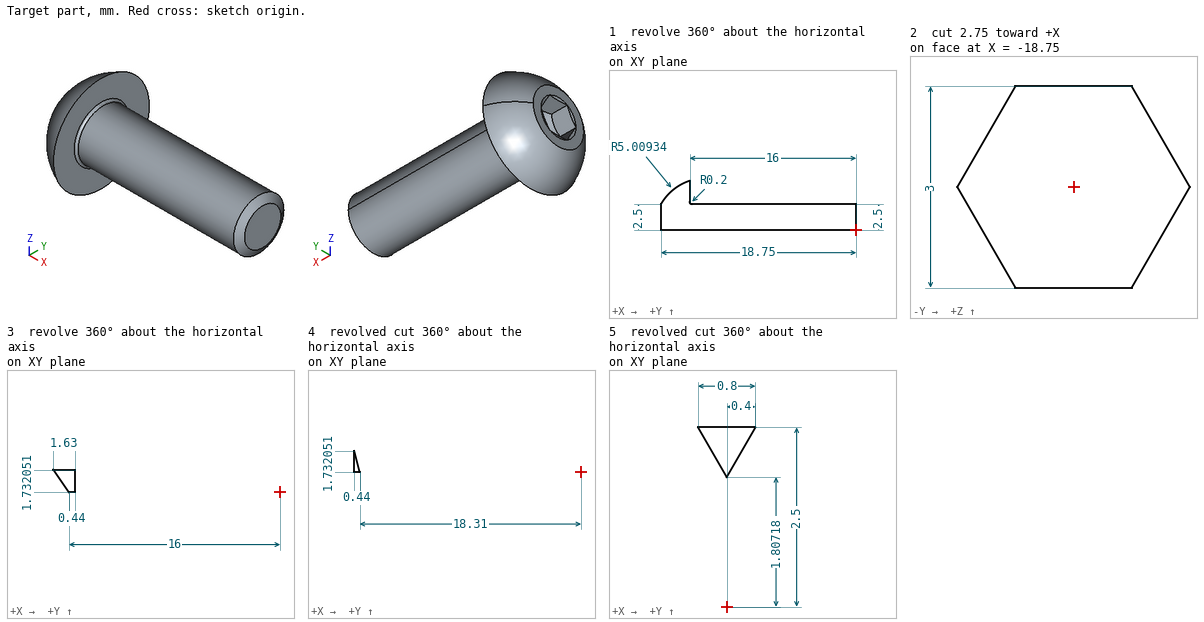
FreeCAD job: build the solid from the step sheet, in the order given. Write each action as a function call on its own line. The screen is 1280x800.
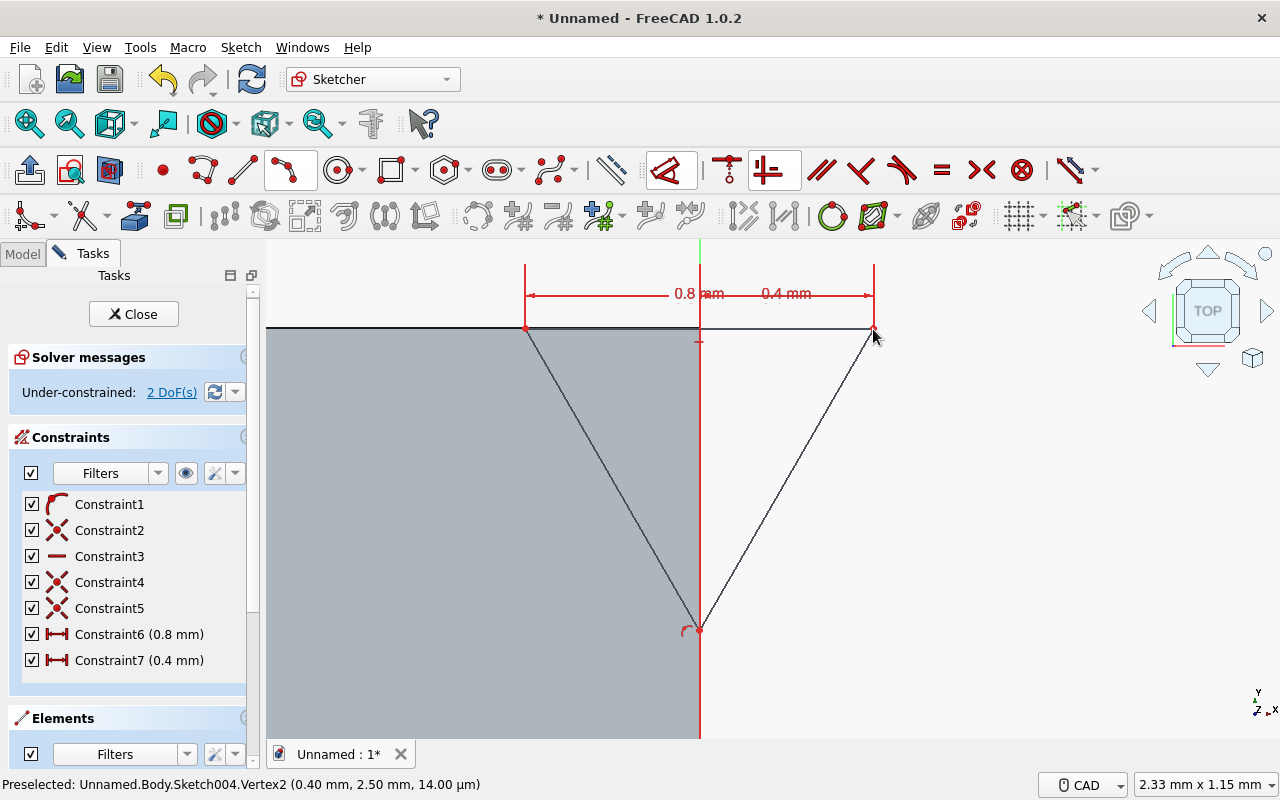
click(874, 329)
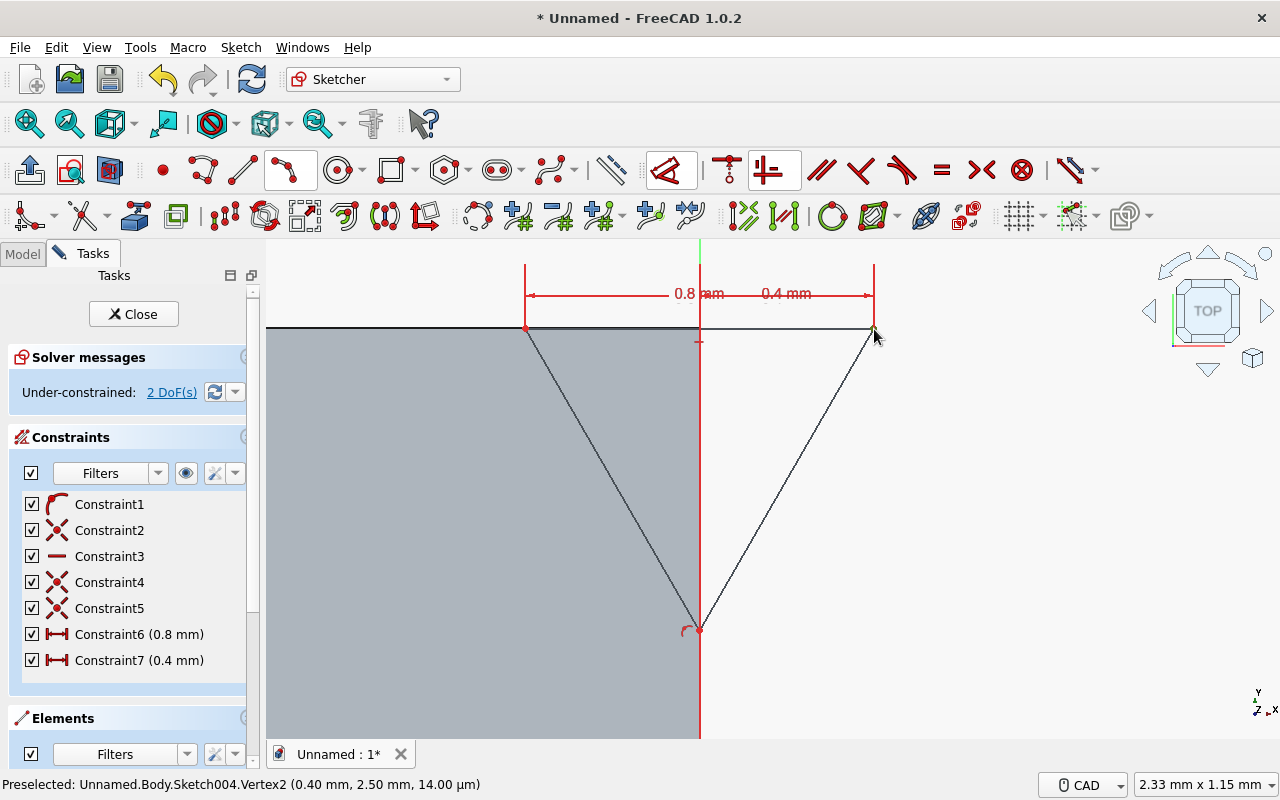
key(i)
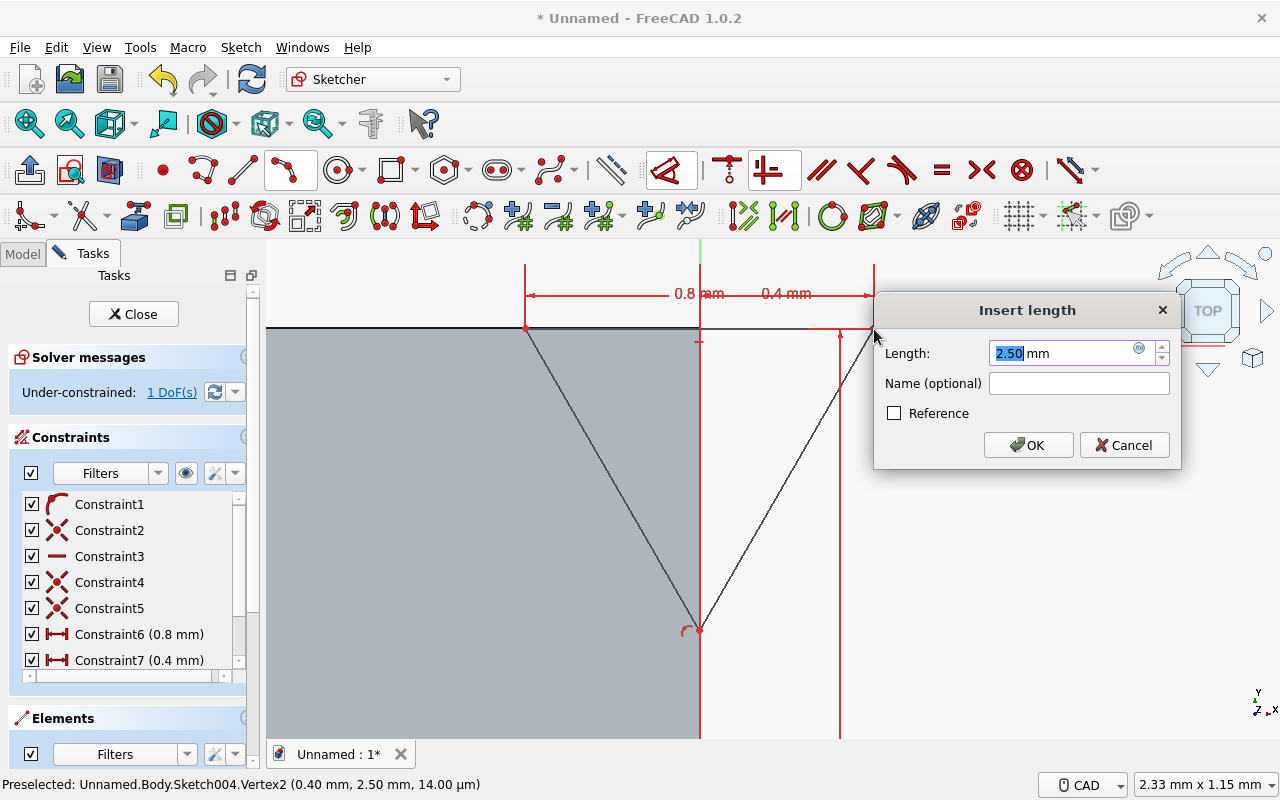
text(2.5)
key(Return)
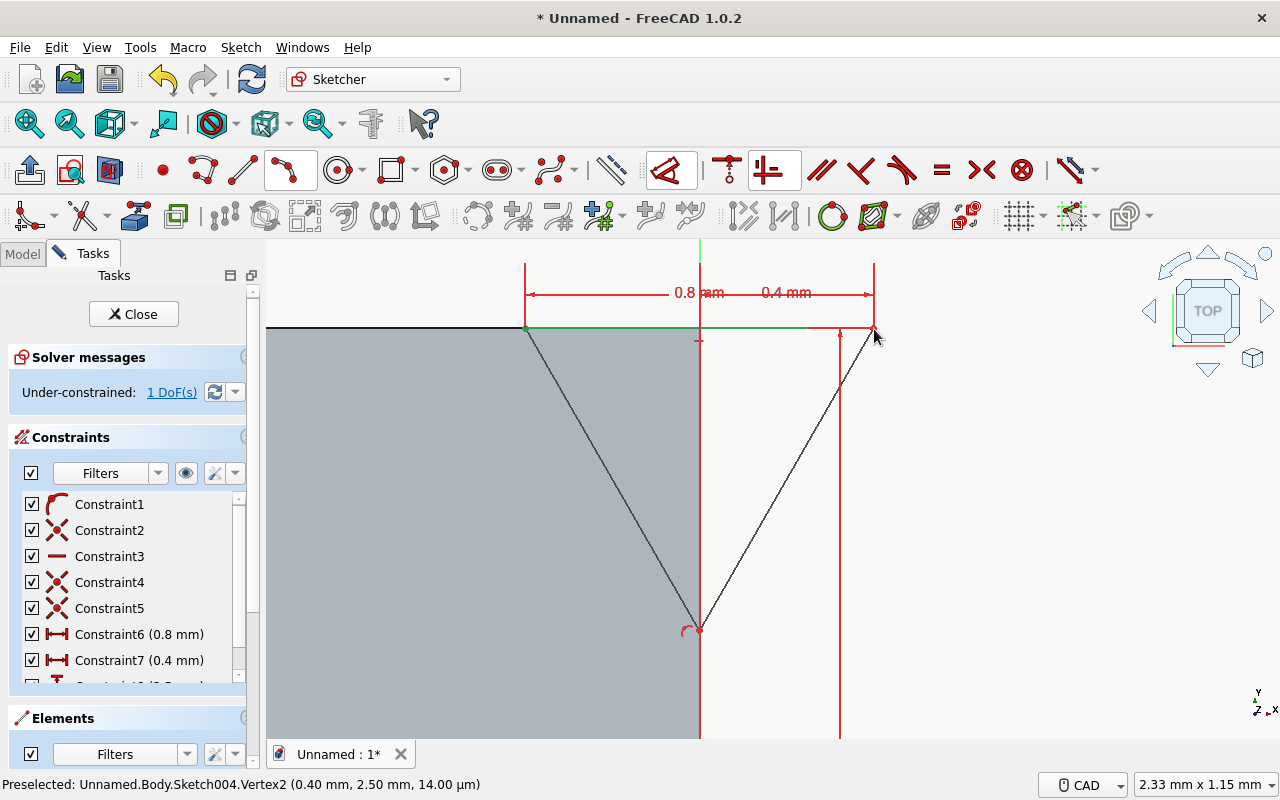
click(700, 631)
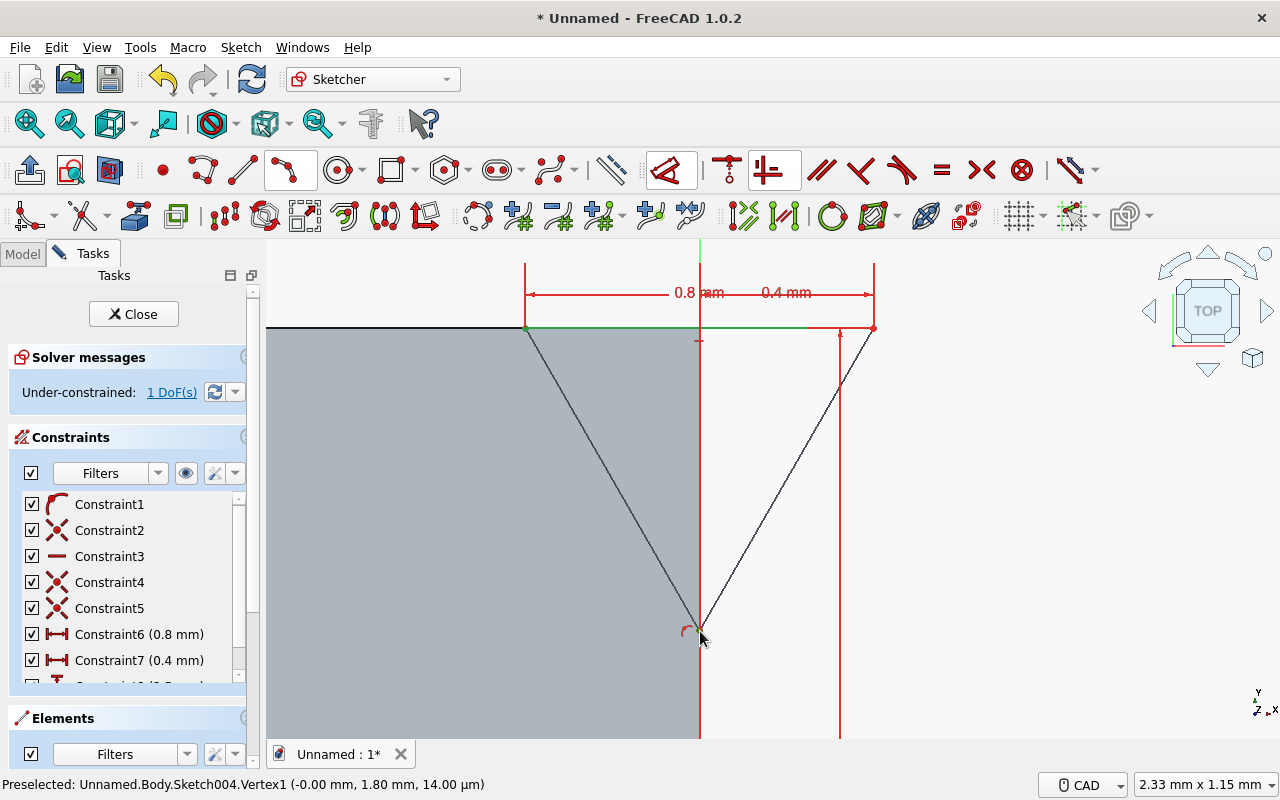
click(692, 170)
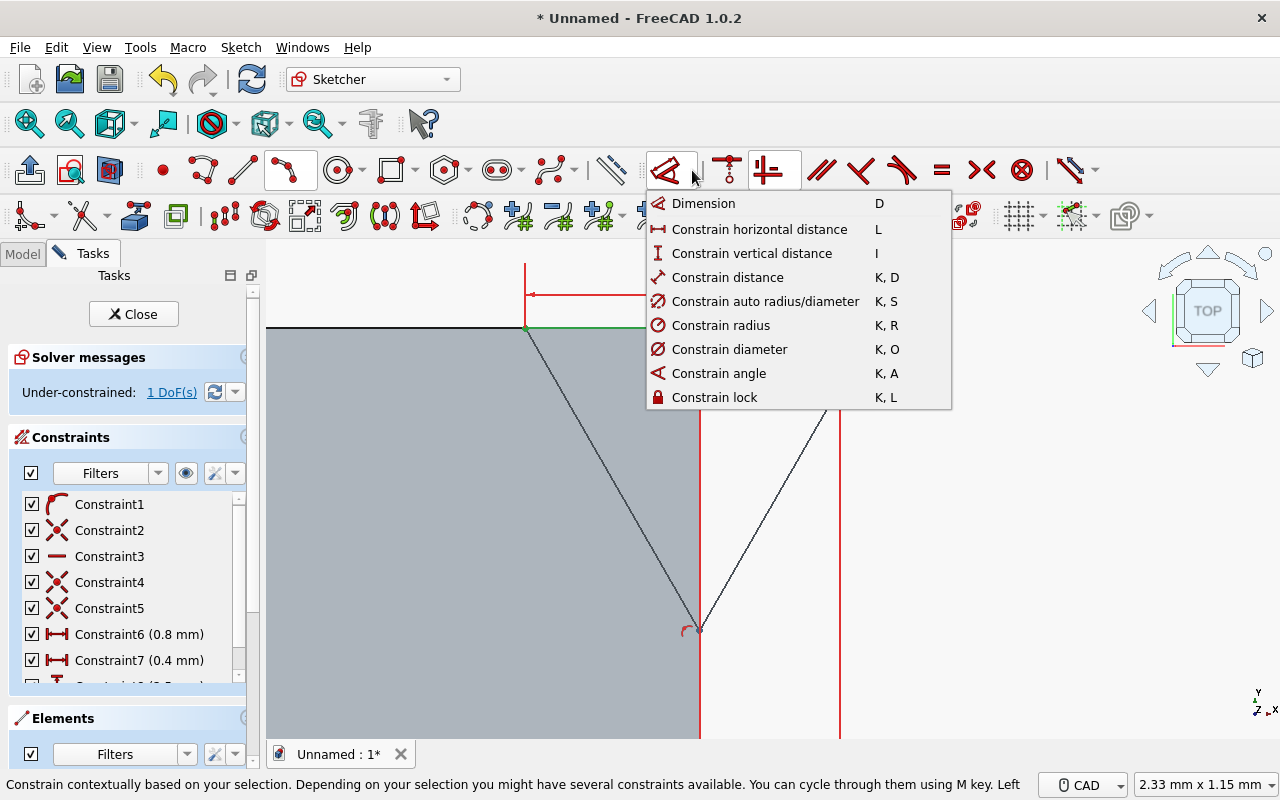
click(799, 253)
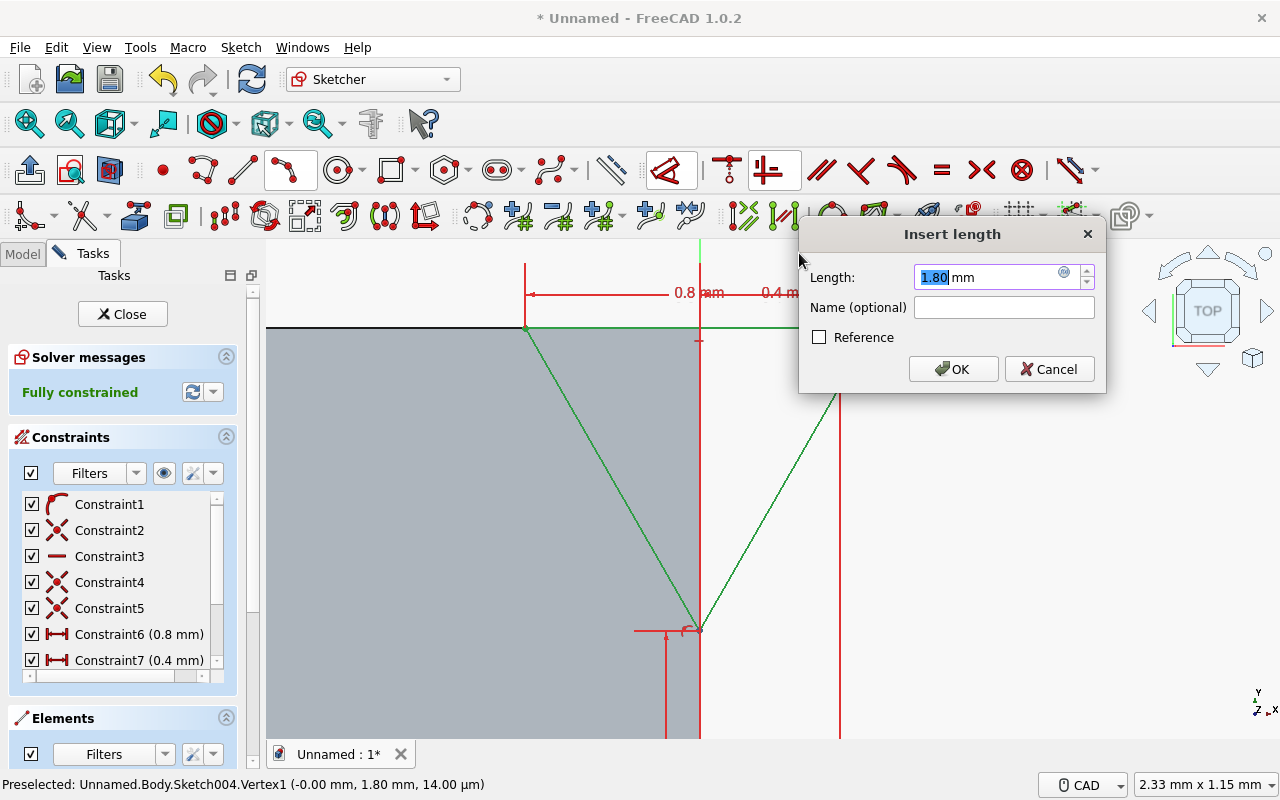
text(1.80718)
key(Return)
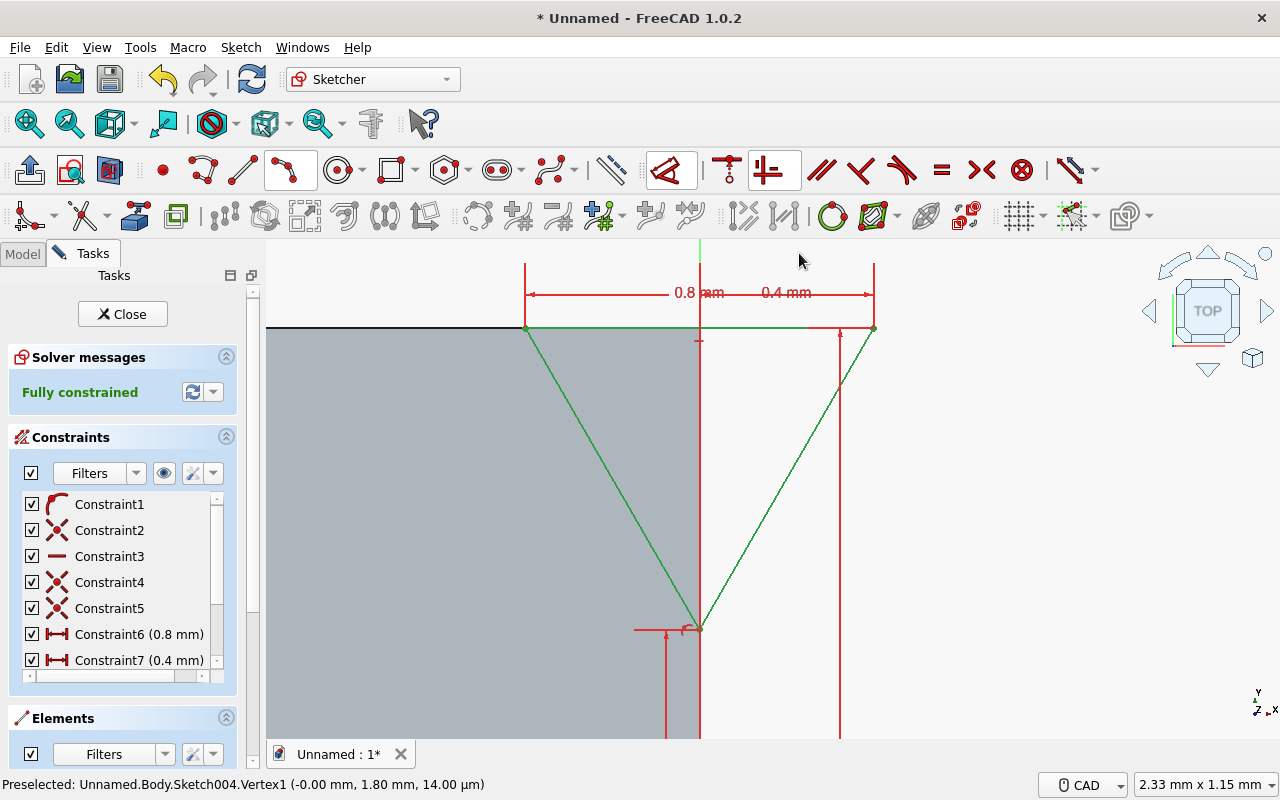
click(123, 314)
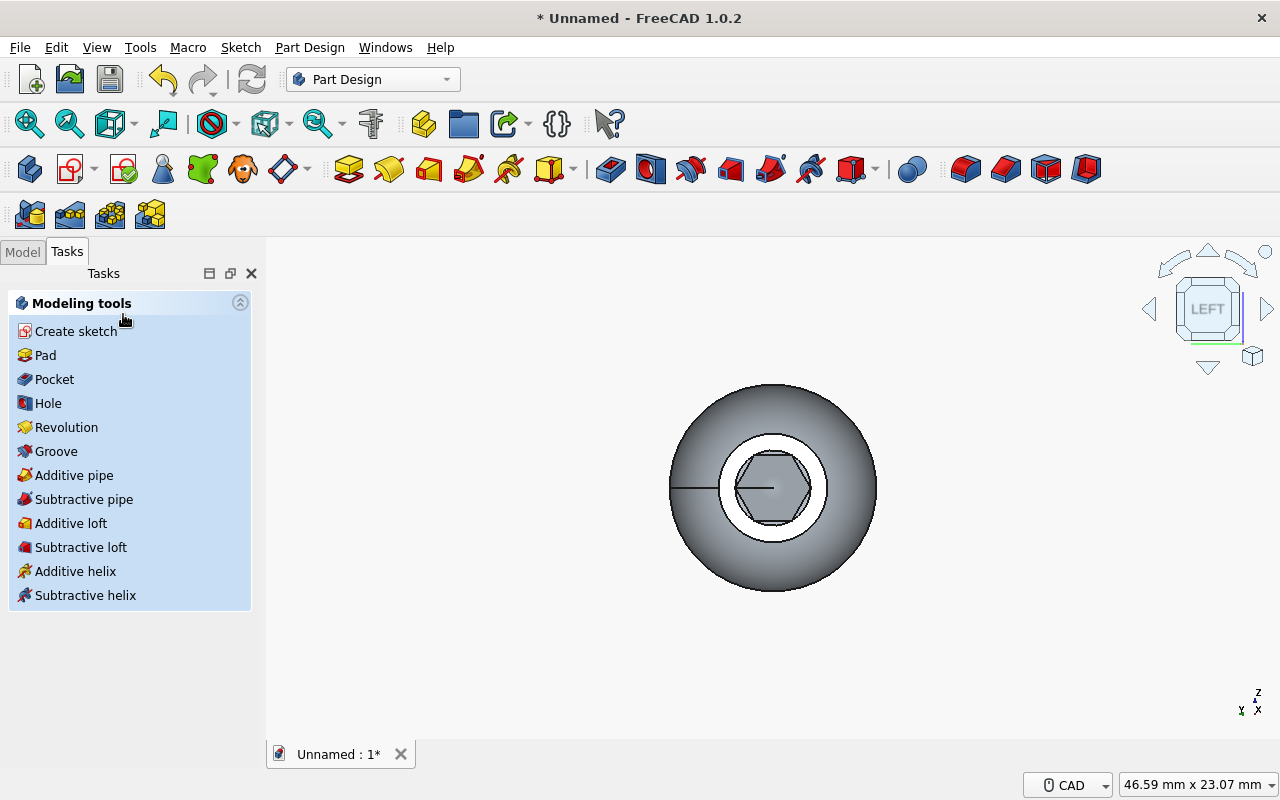
click(692, 170)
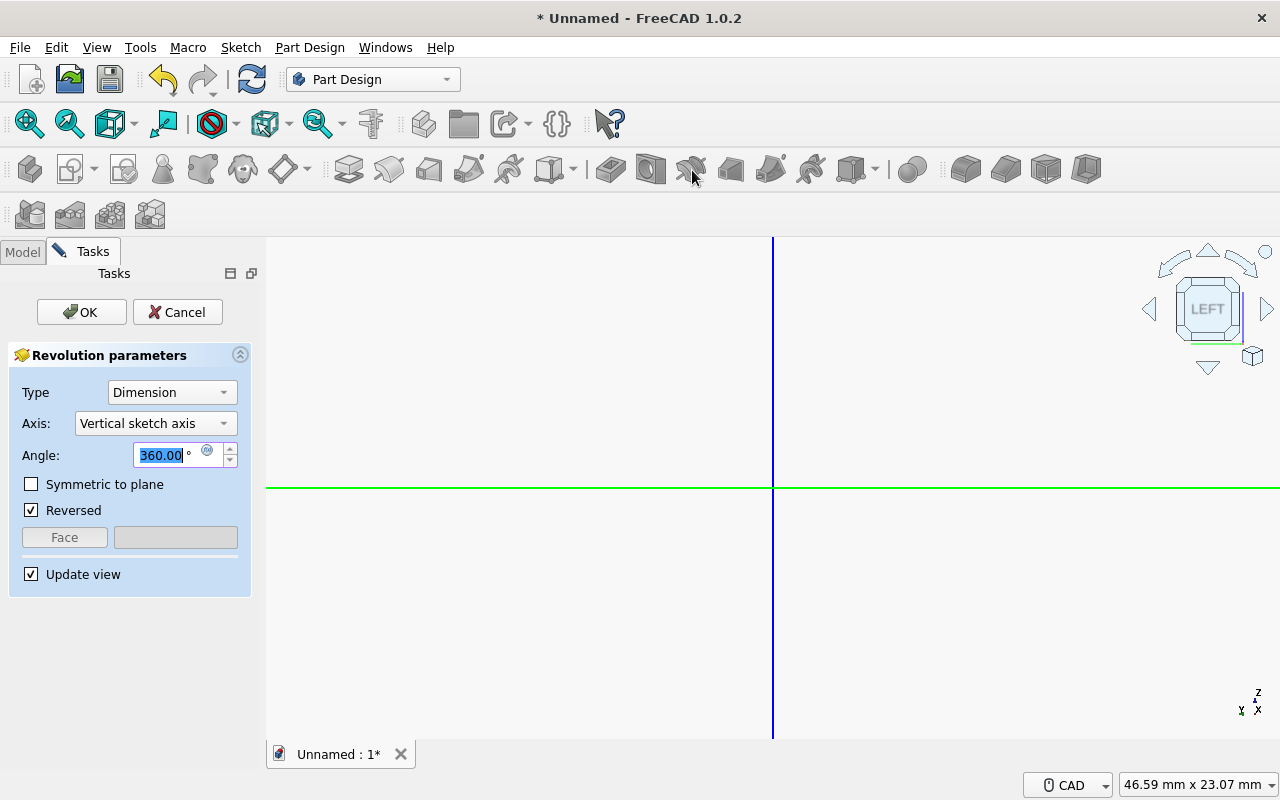
click(156, 424)